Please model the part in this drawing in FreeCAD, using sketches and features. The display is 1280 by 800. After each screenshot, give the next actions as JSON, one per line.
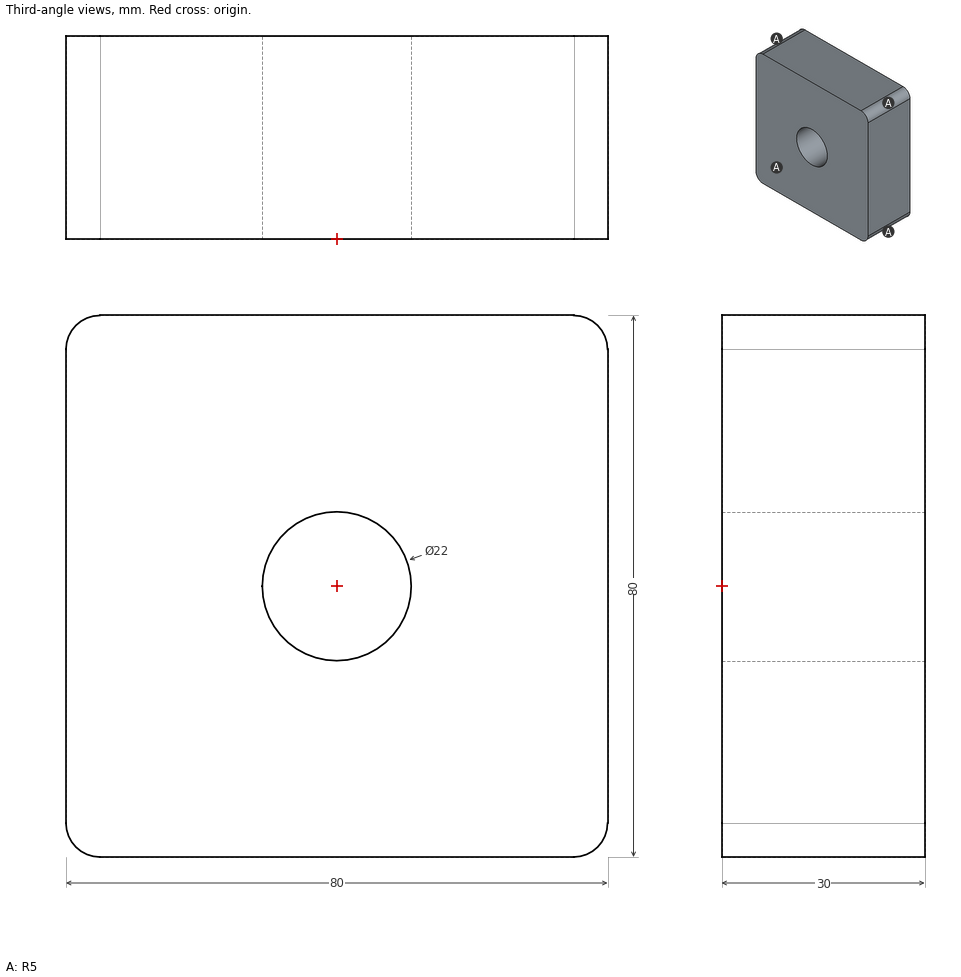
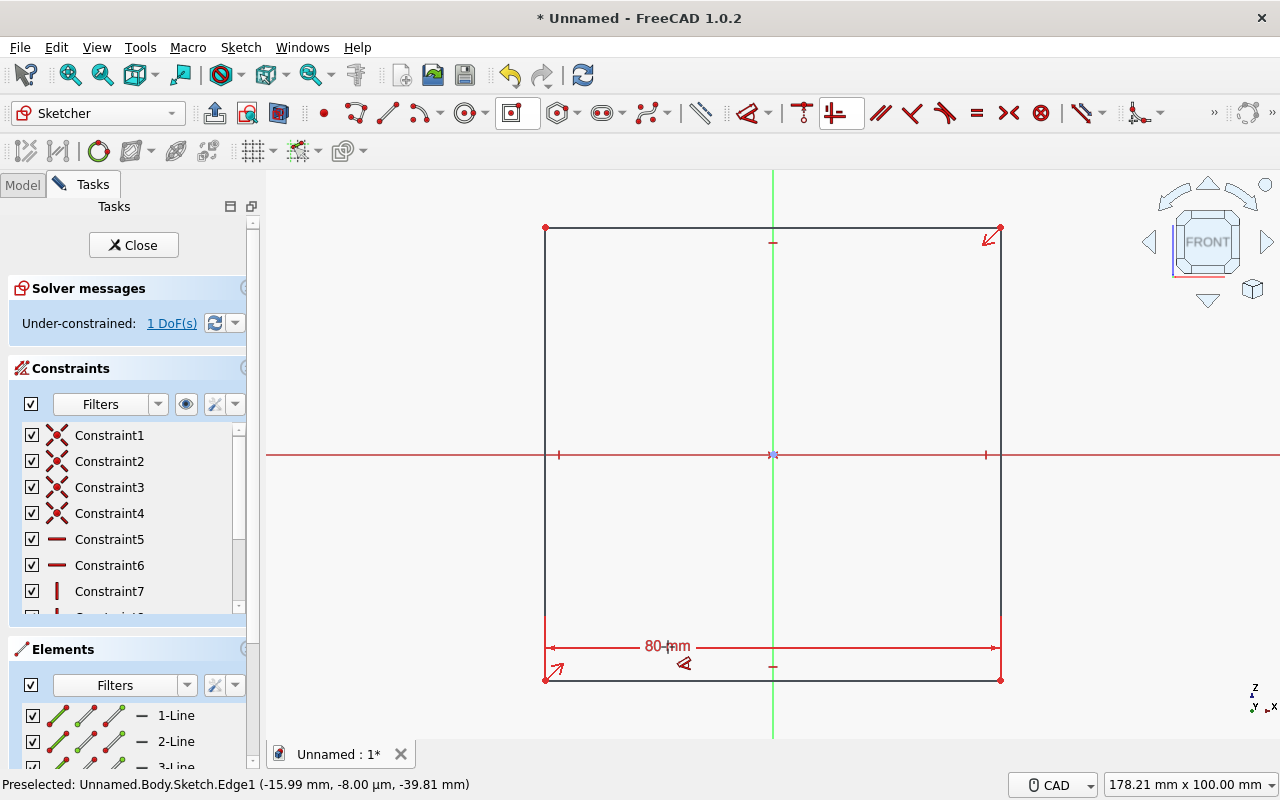
{"action": "left_click", "coordinate": [1001, 545]}
{"action": "left_click", "coordinate": [1035, 350]}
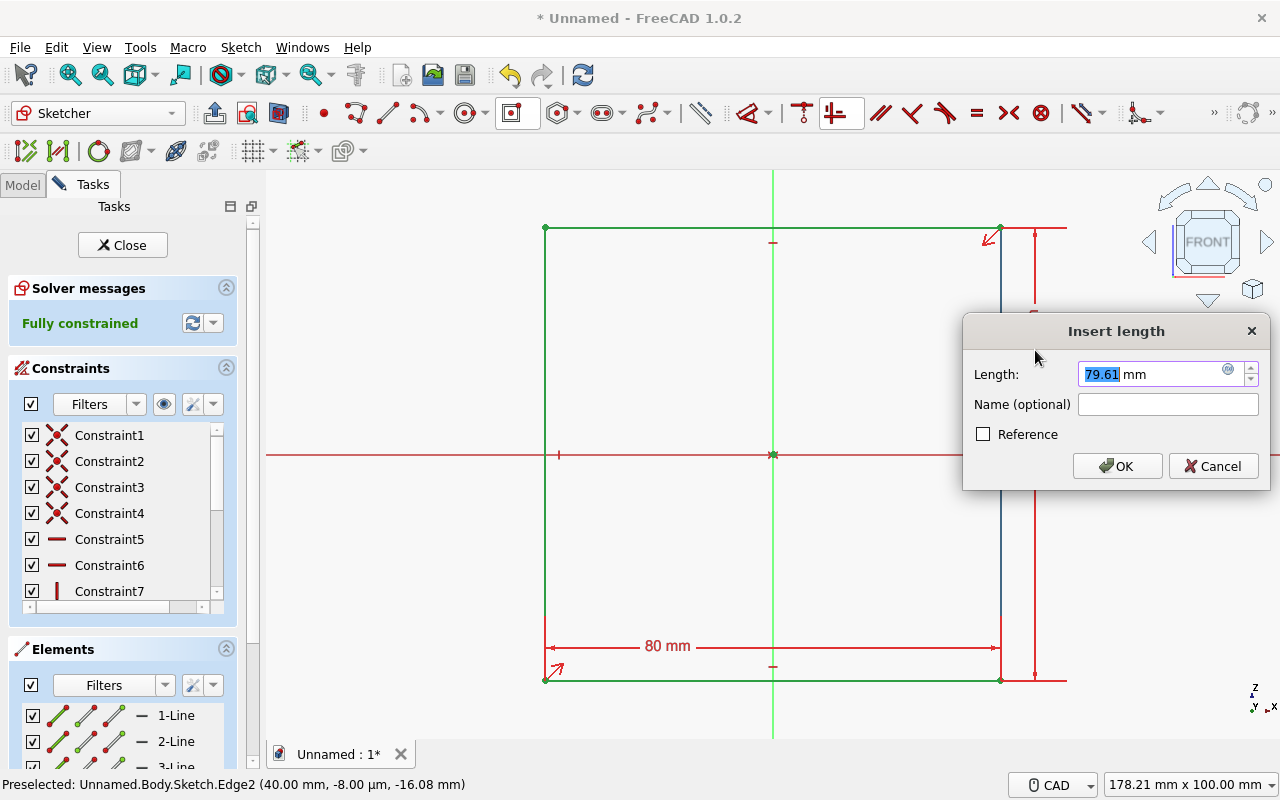
{"action": "type", "text": "80"}
{"action": "key", "text": "Return"}
{"action": "key", "text": "Escape"}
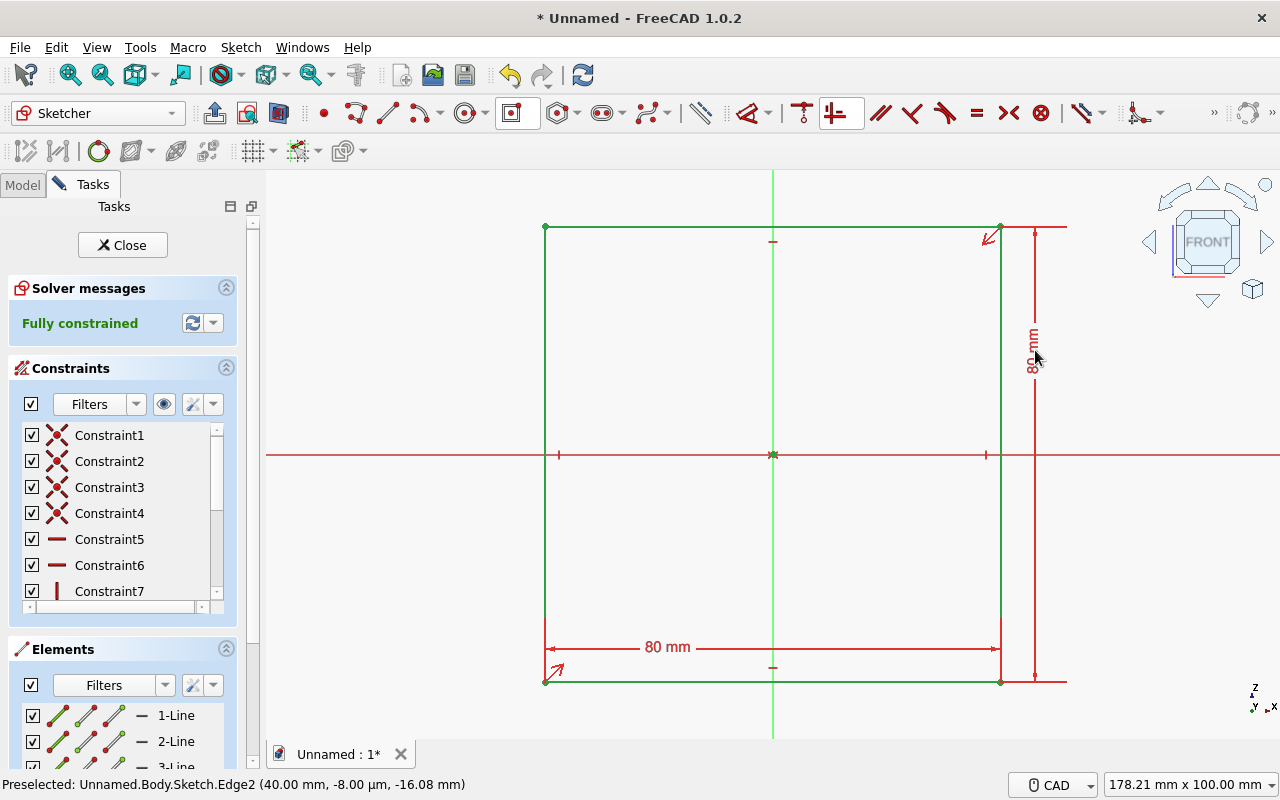
{"action": "left_click", "coordinate": [123, 245]}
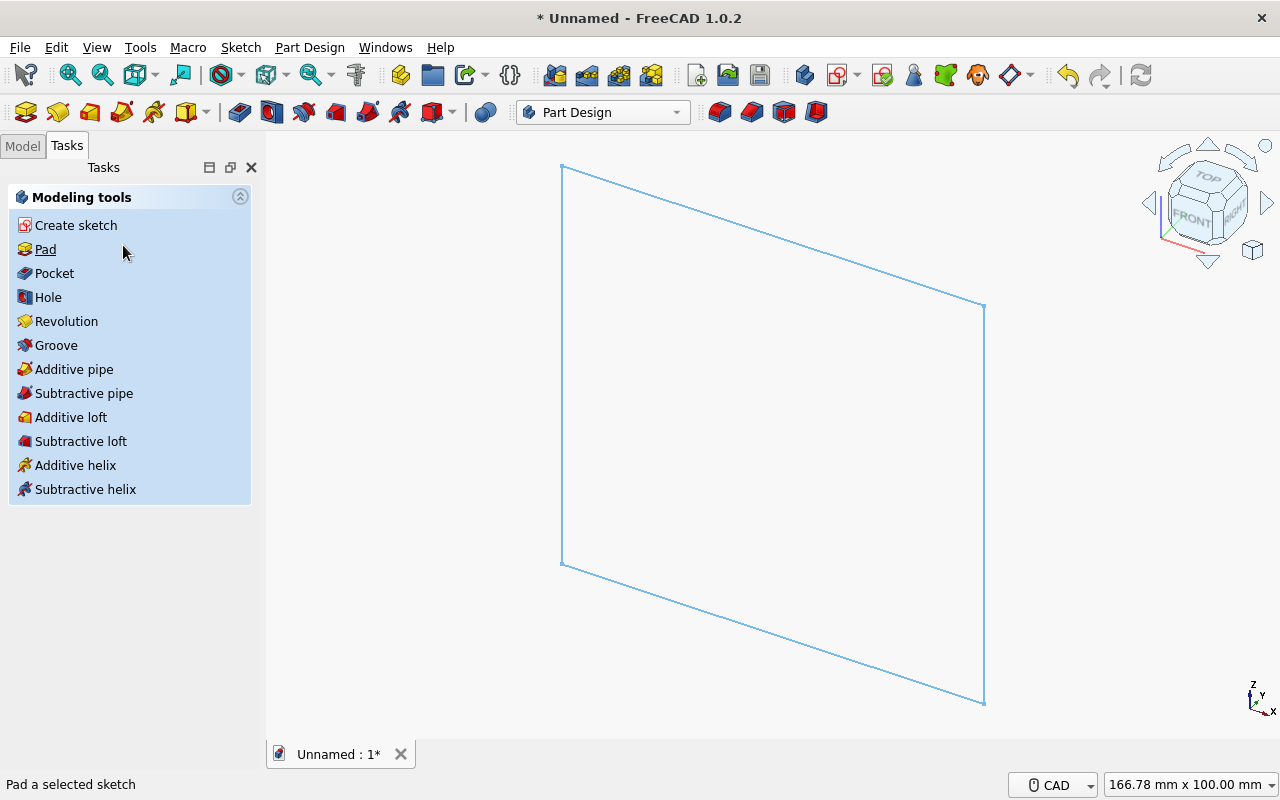
{"action": "left_click", "coordinate": [26, 112]}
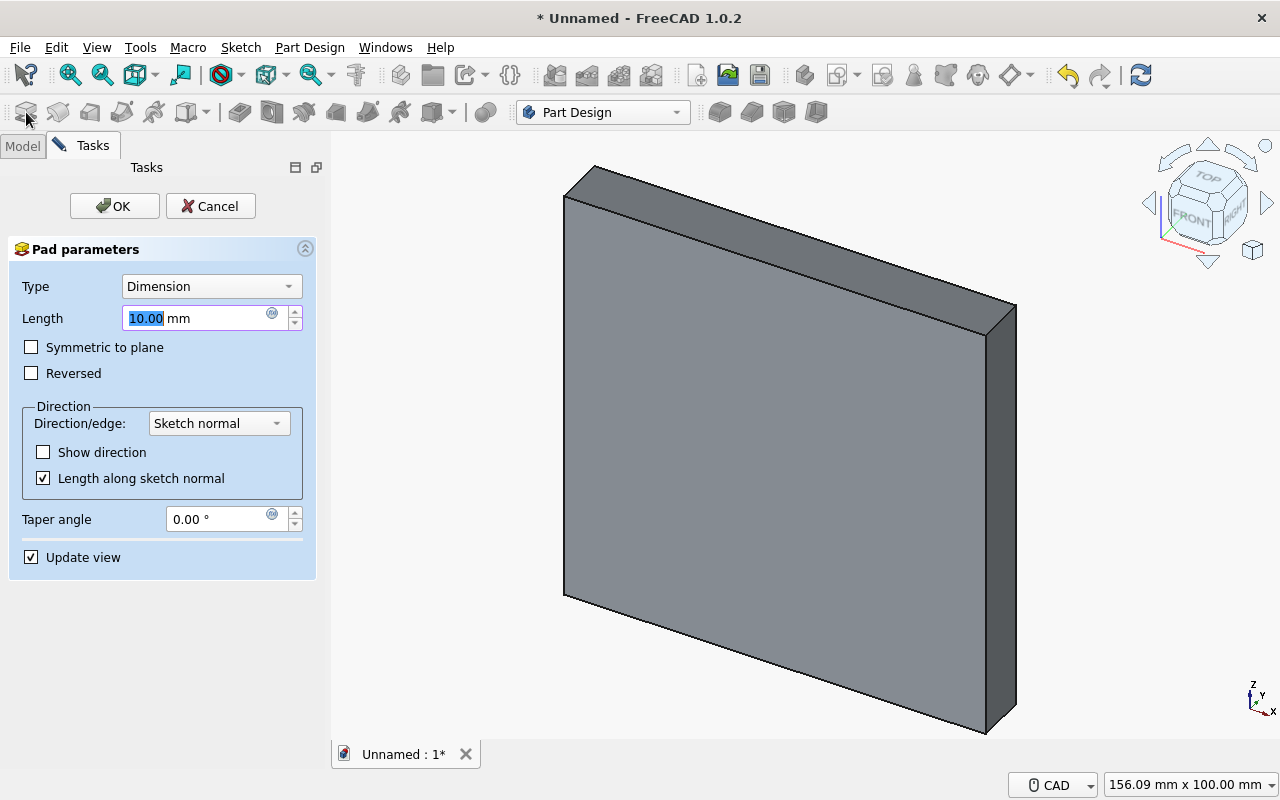
{"action": "type", "text": "30"}
{"action": "key", "text": "Tab"}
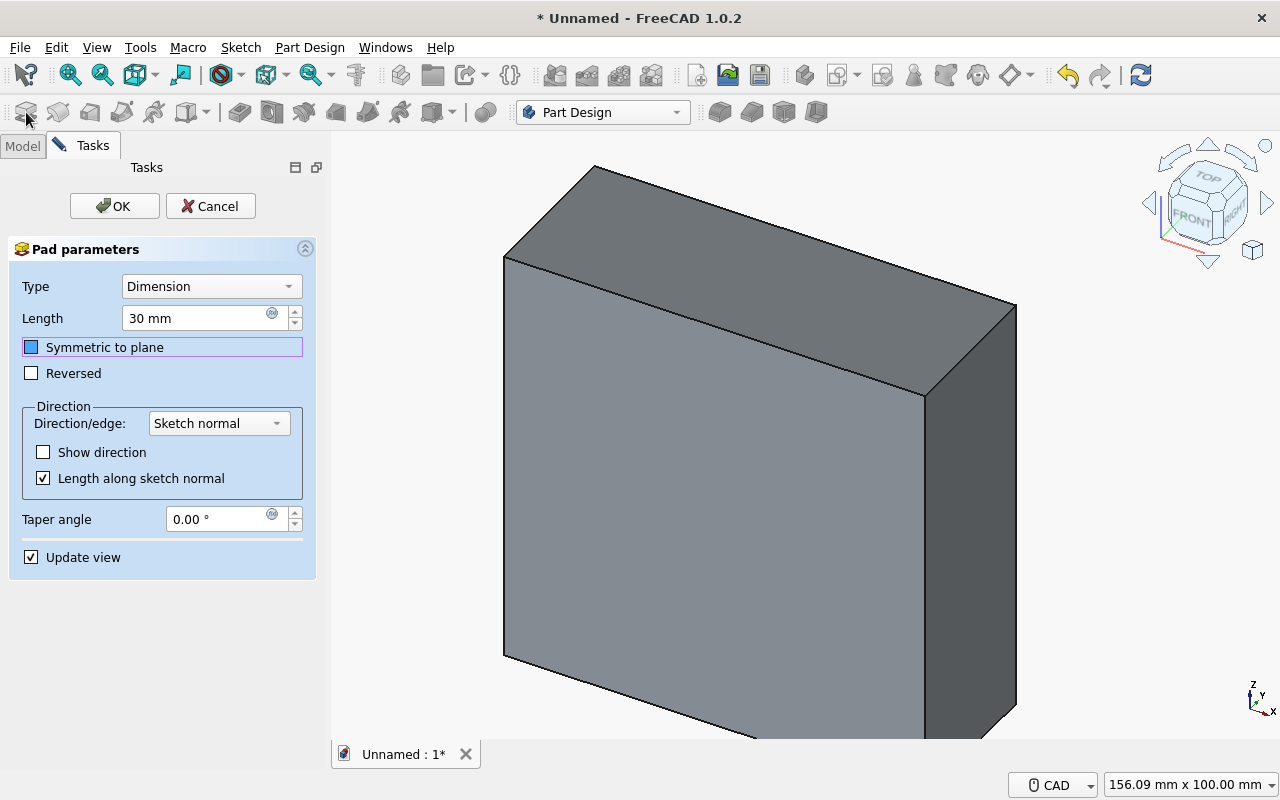
{"action": "left_click", "coordinate": [30, 373]}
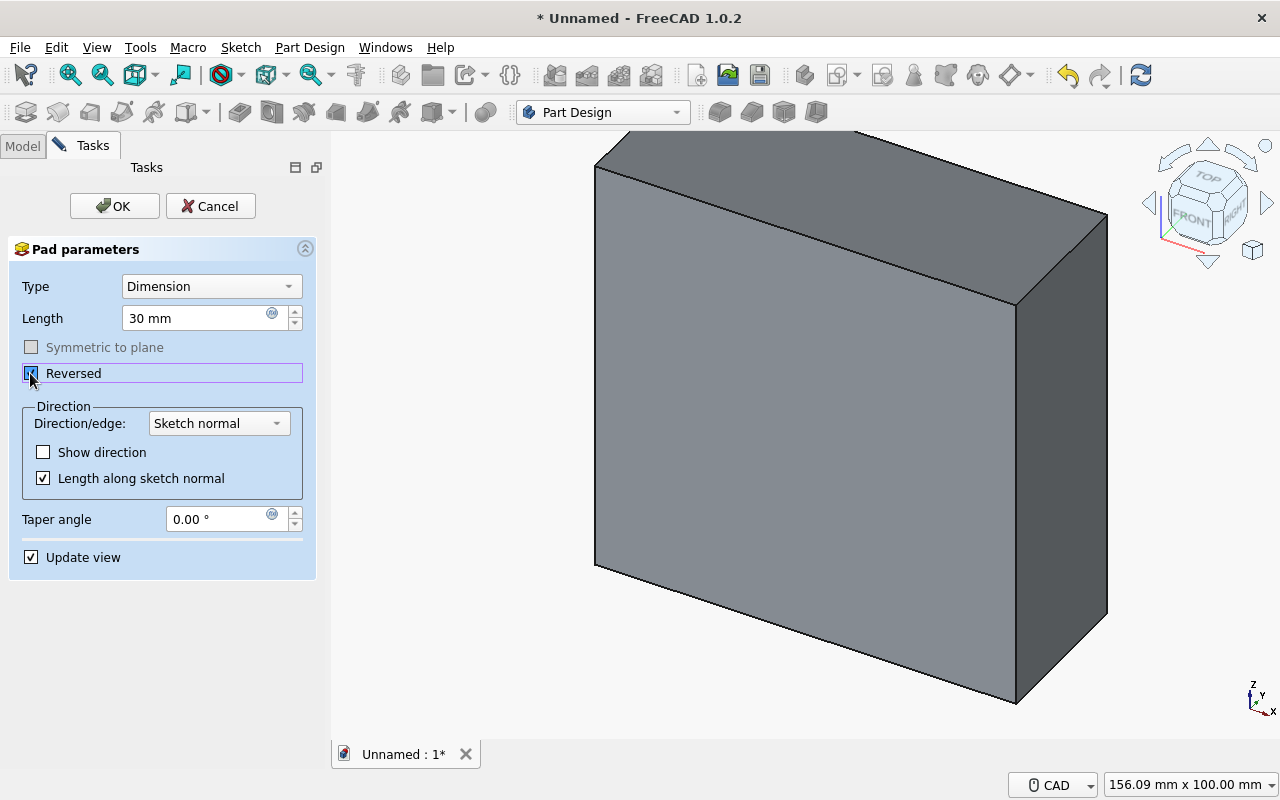
{"action": "left_click", "coordinate": [115, 206]}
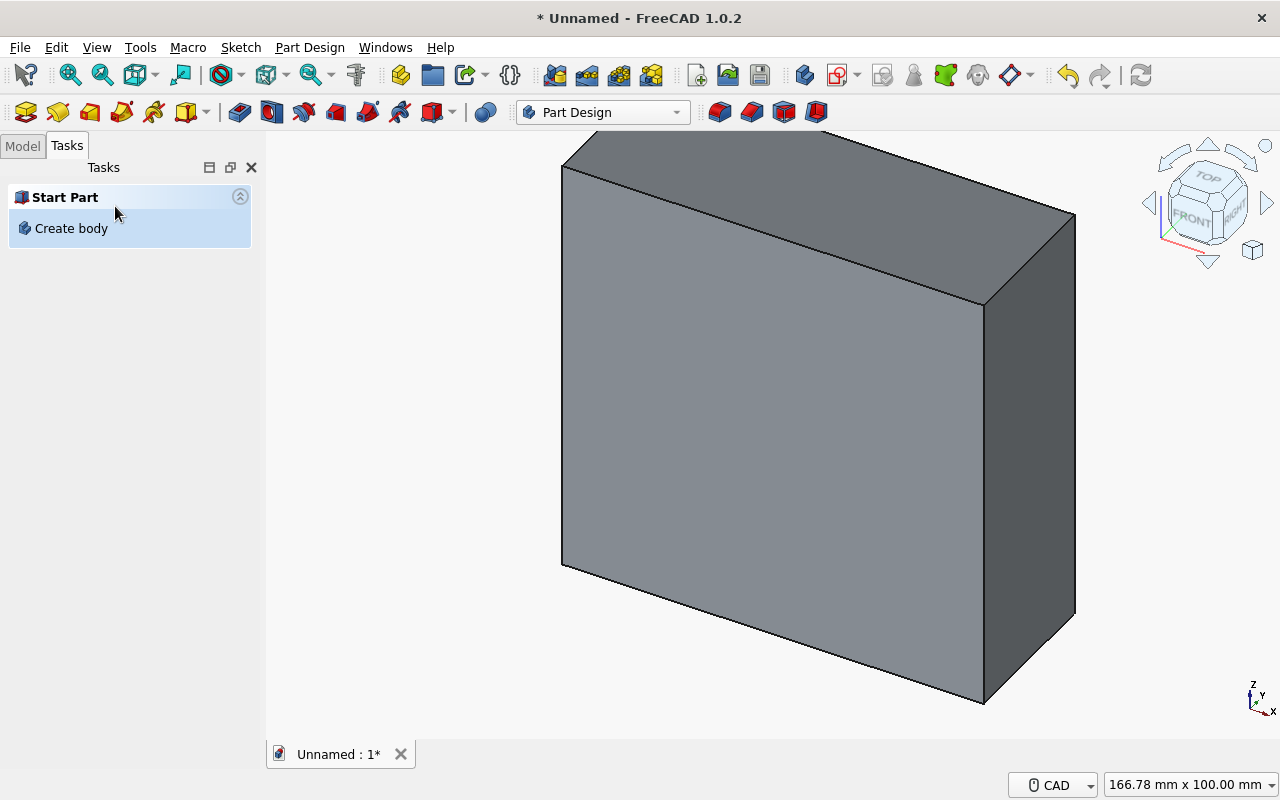
{"action": "left_click", "coordinate": [72, 76]}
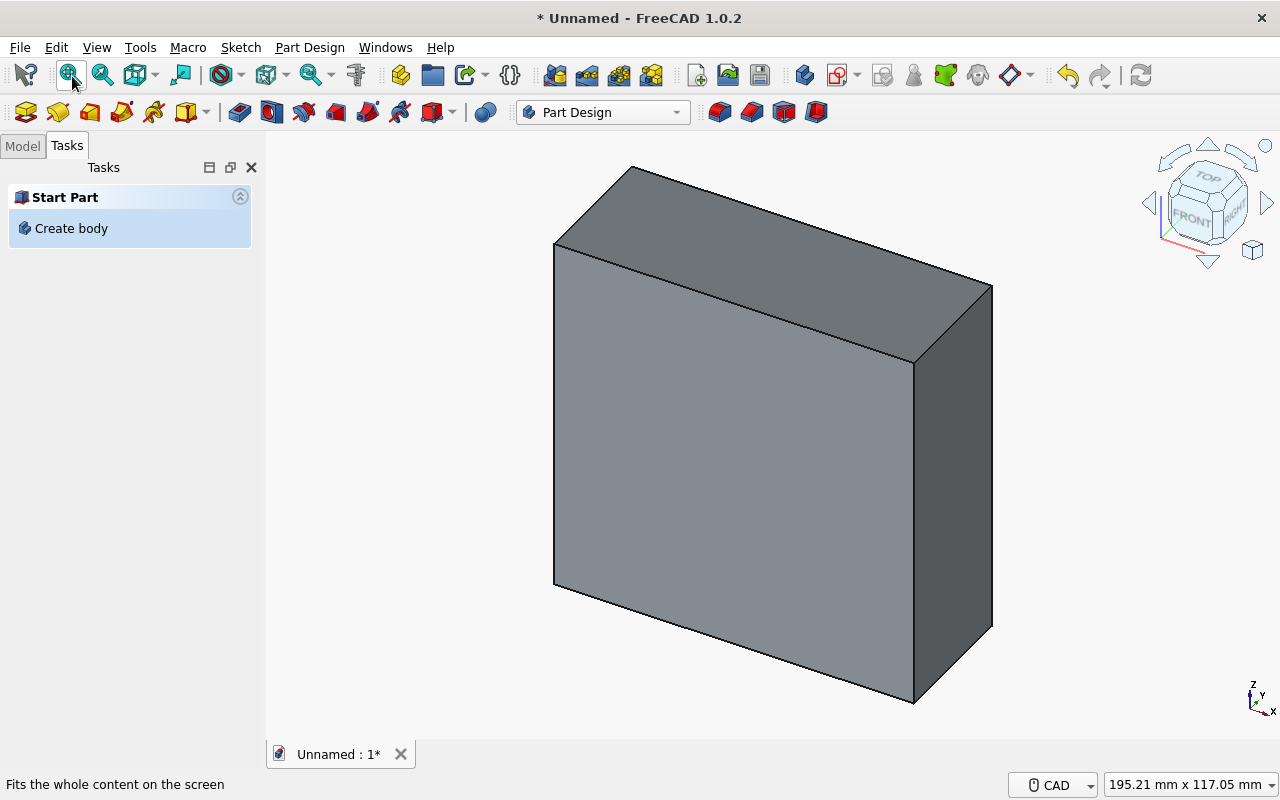
{"action": "left_click", "coordinate": [953, 323]}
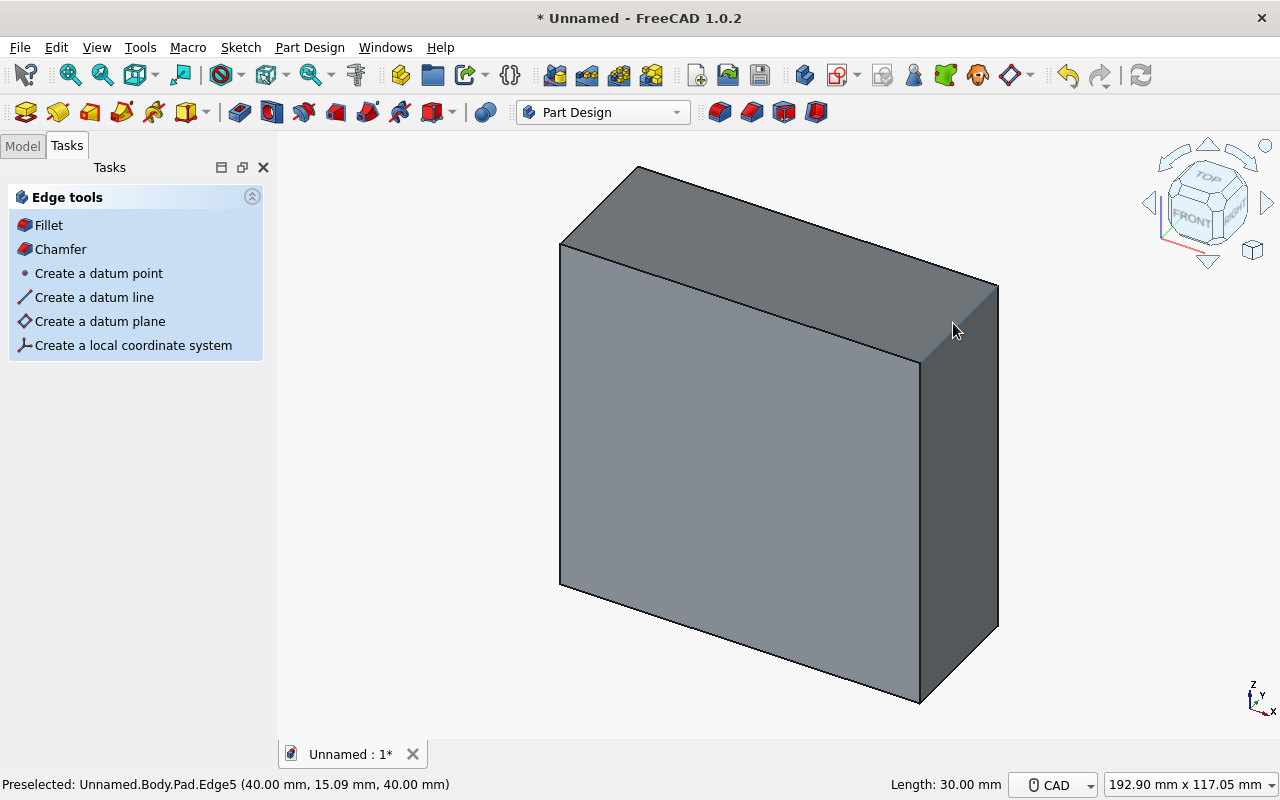
{"action": "key", "text": "0"}